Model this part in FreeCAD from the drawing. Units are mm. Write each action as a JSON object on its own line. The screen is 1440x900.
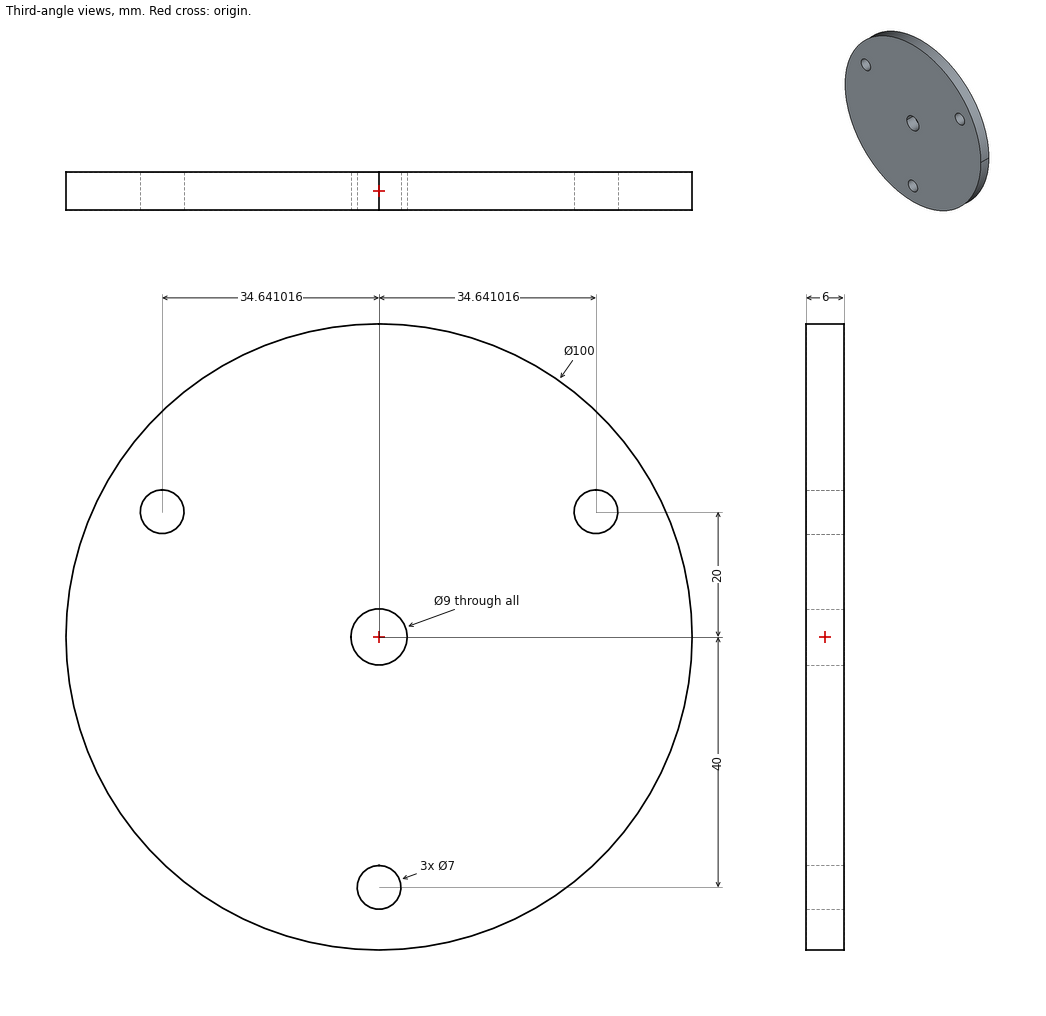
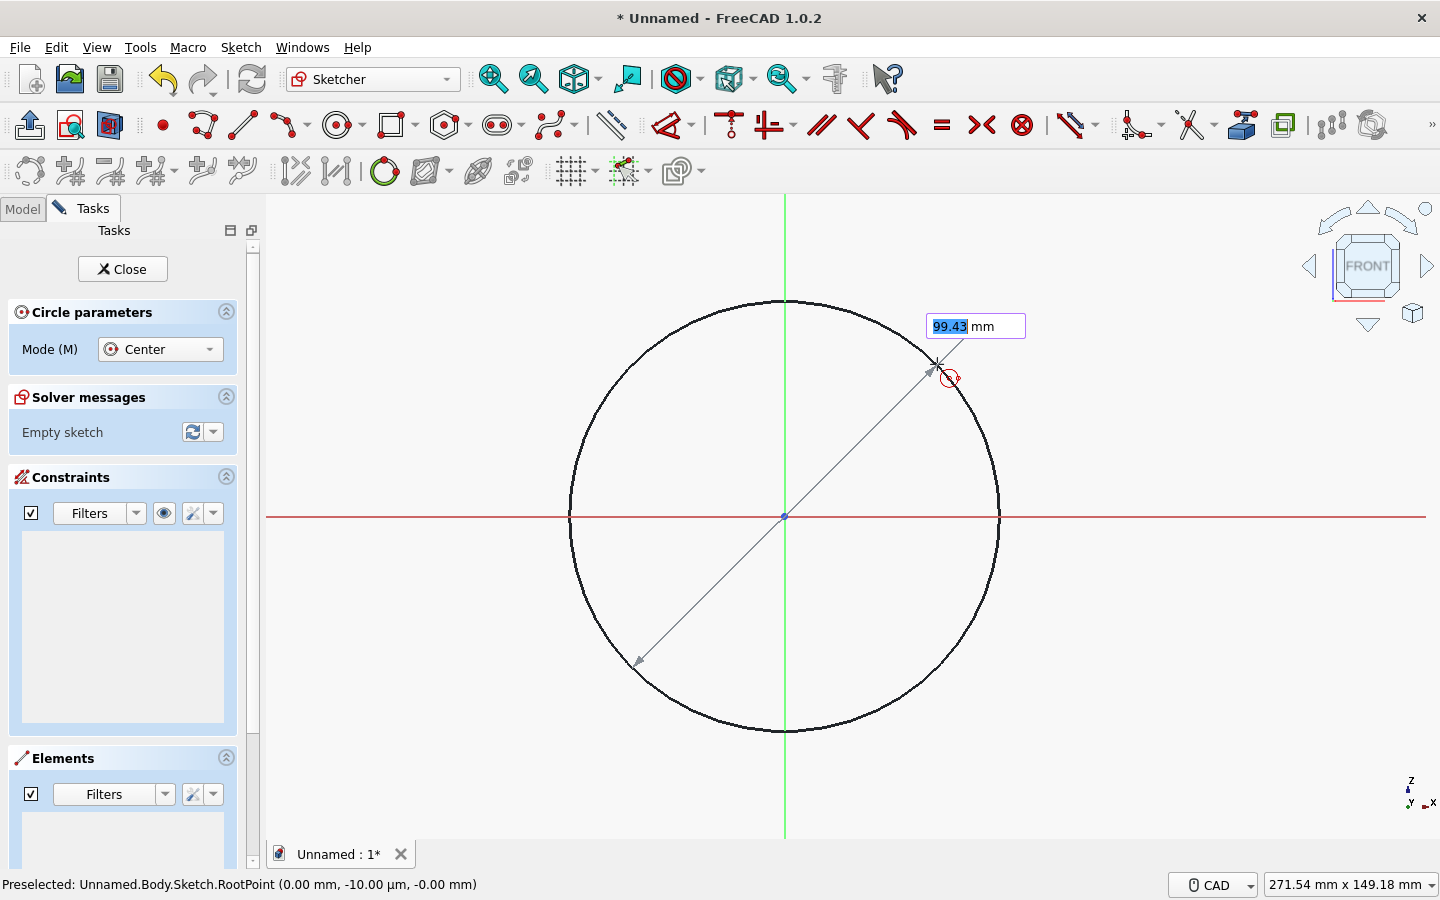
{"action": "type", "text": "100"}
{"action": "key", "text": "Return"}
{"action": "key", "text": "Escape"}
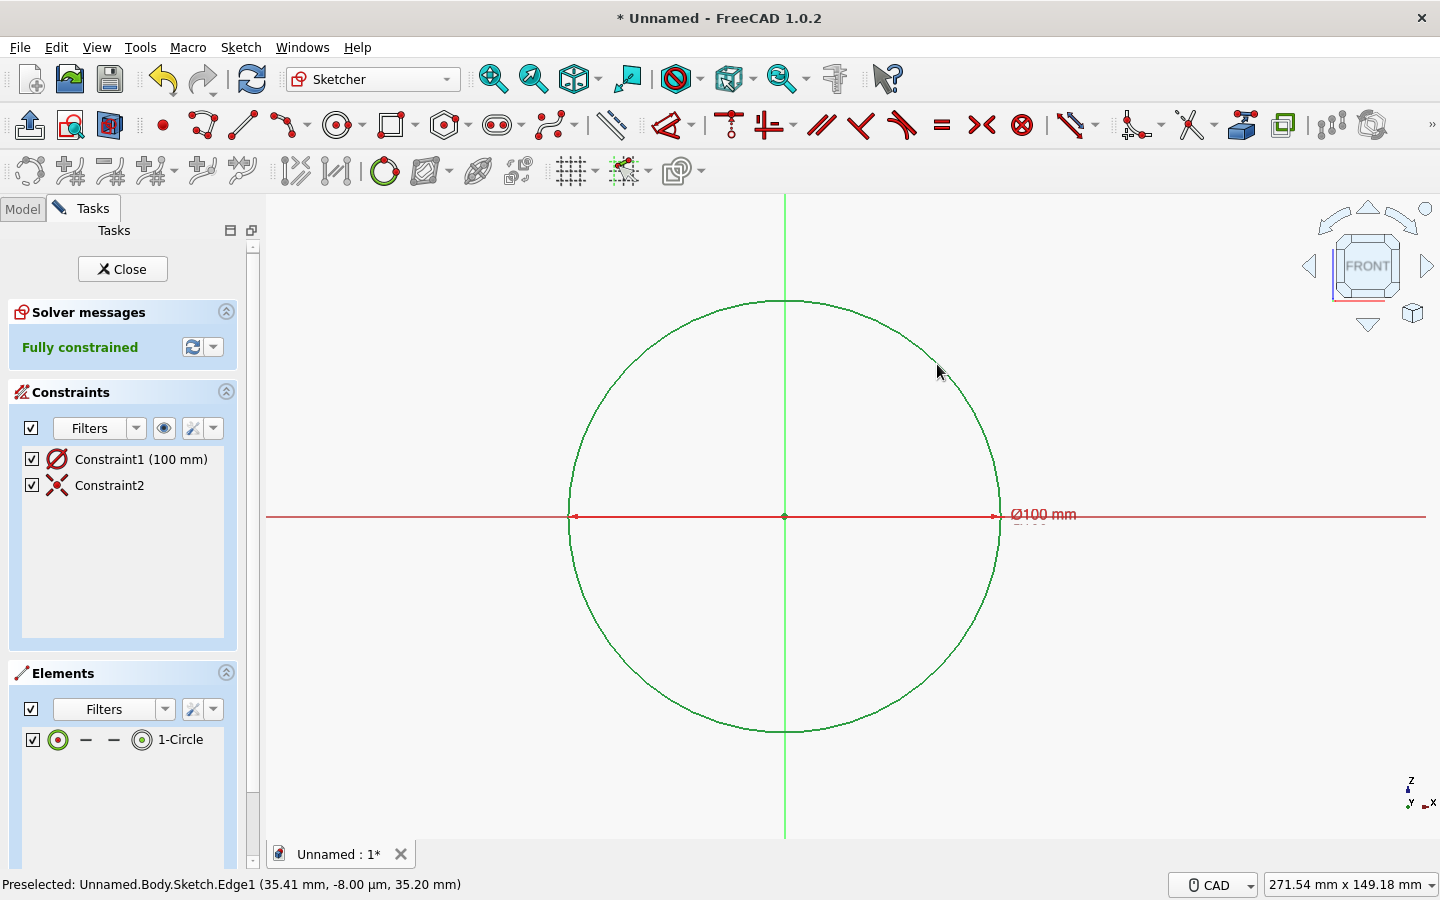
{"action": "left_click", "coordinate": [123, 269]}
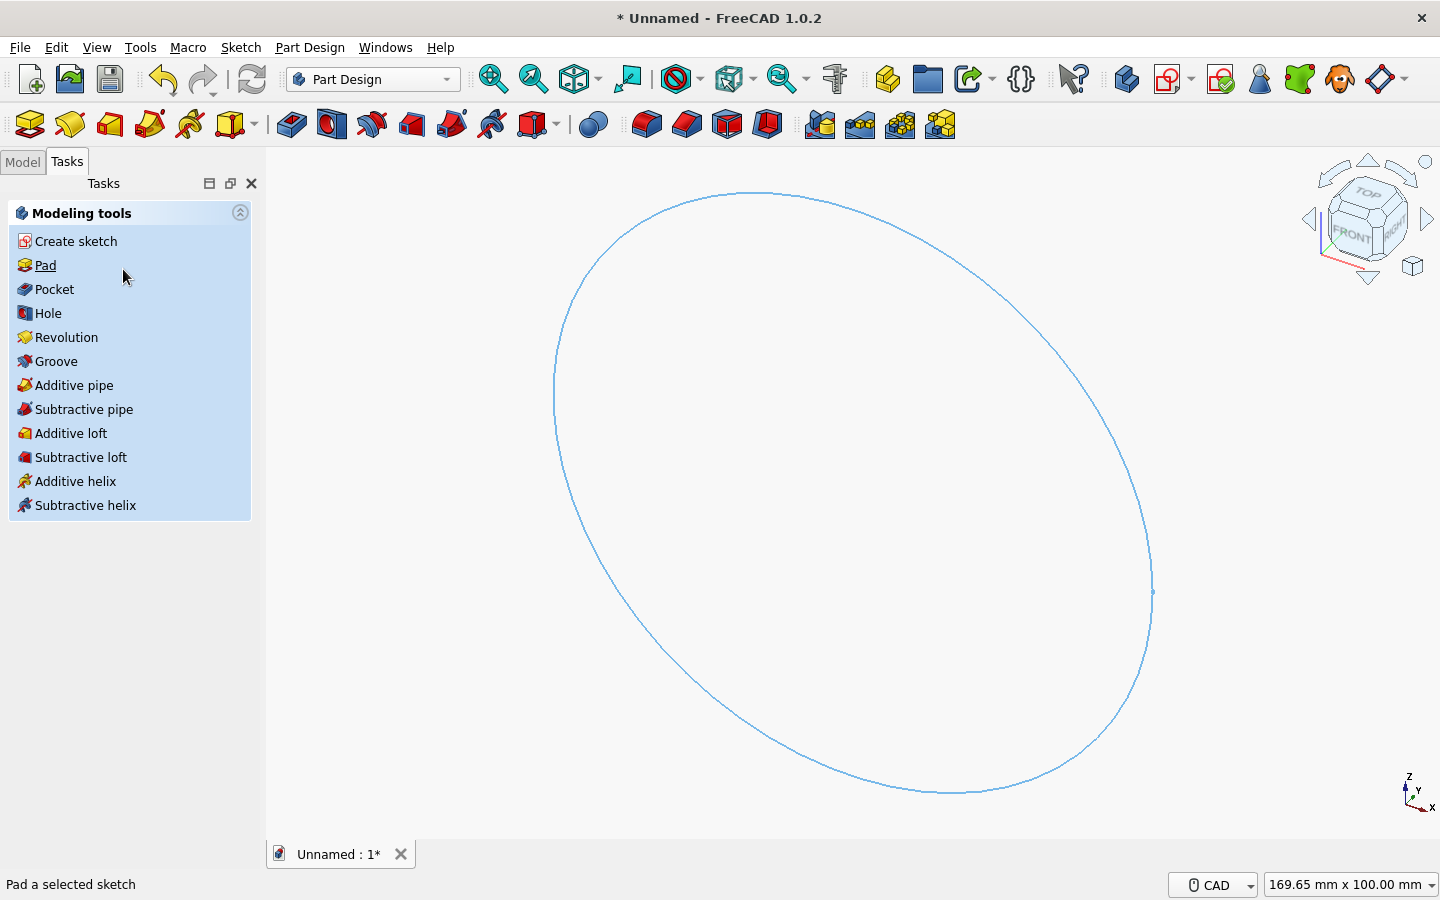
{"action": "left_click", "coordinate": [30, 124]}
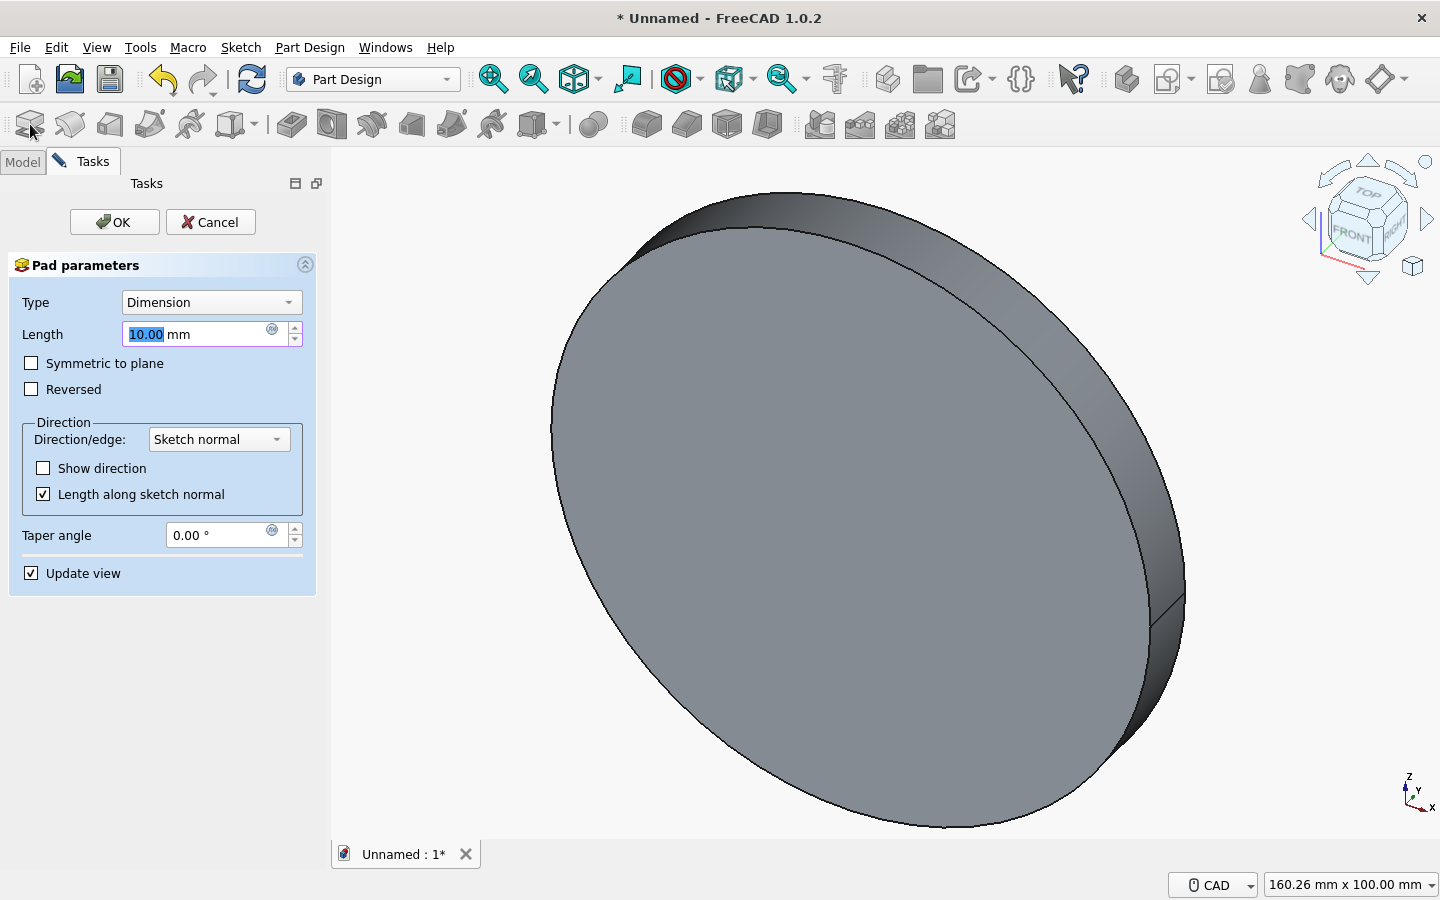
{"action": "type", "text": "6"}
{"action": "key", "text": "Tab"}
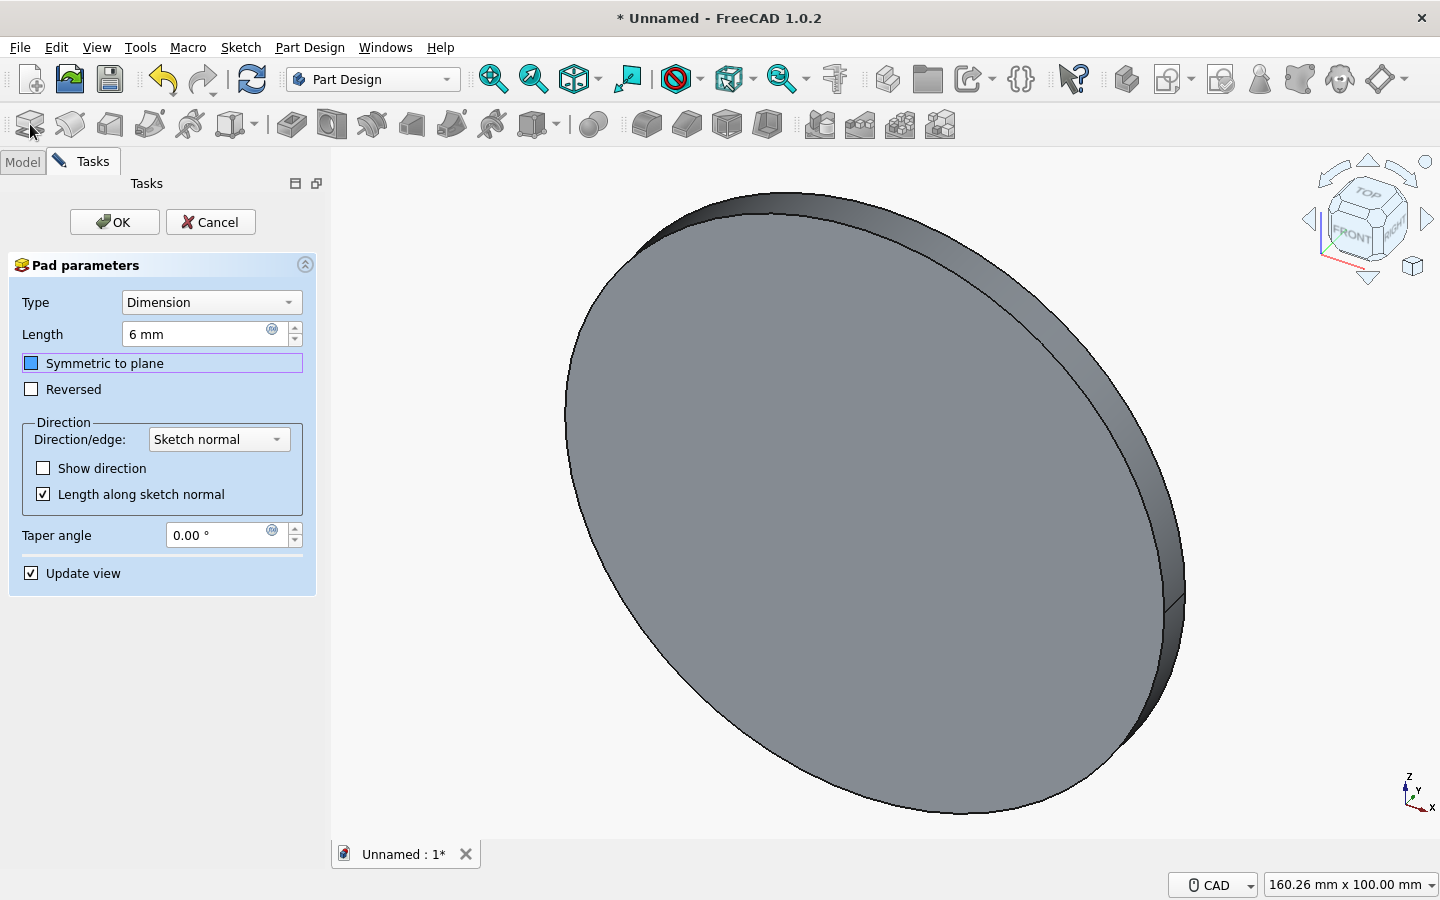
{"action": "left_click", "coordinate": [30, 363]}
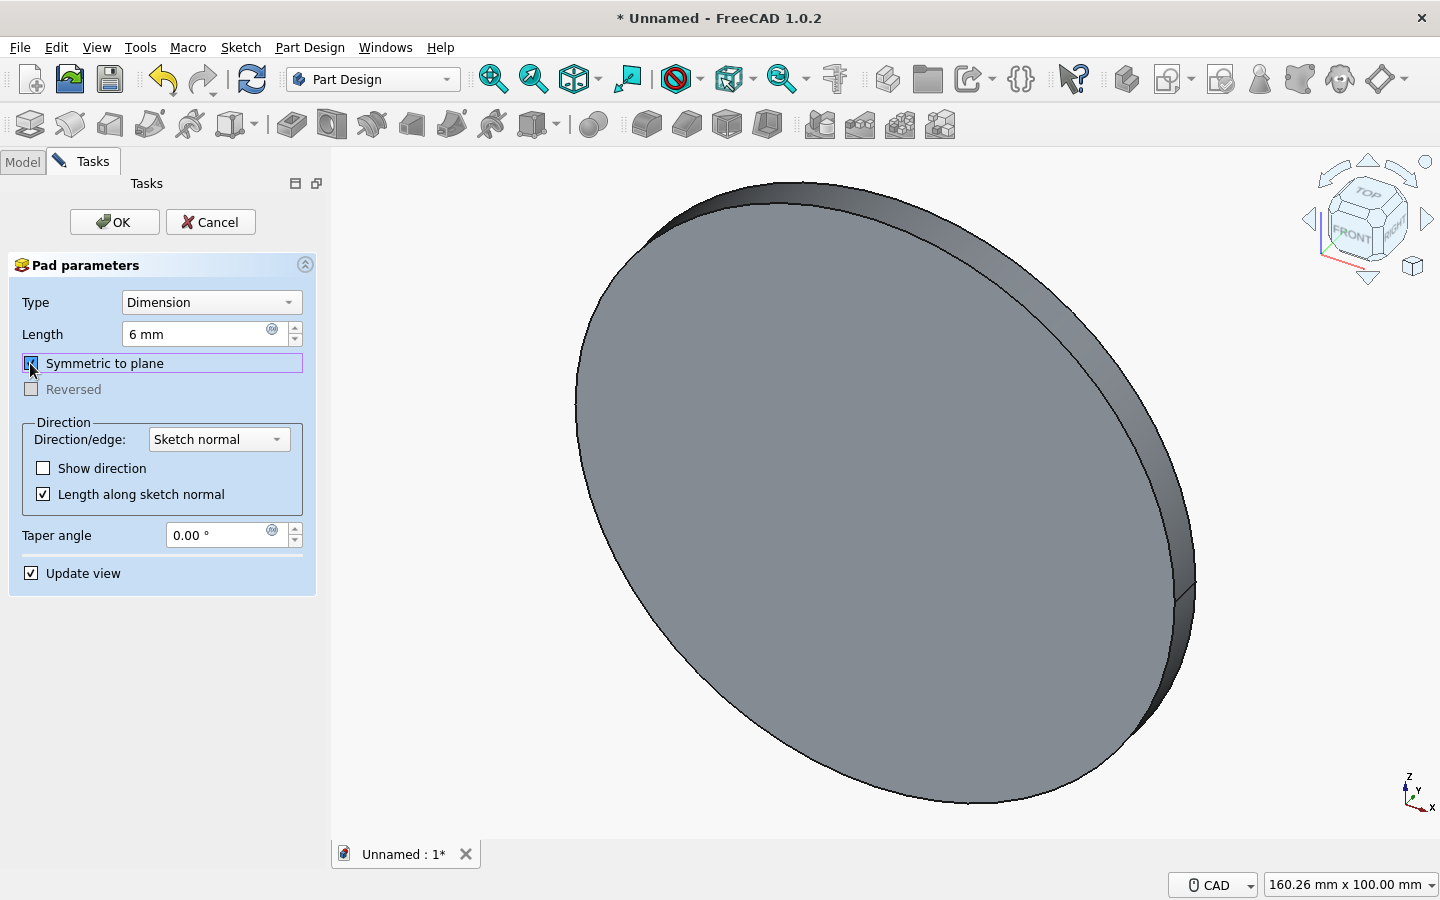
{"action": "left_click", "coordinate": [115, 222]}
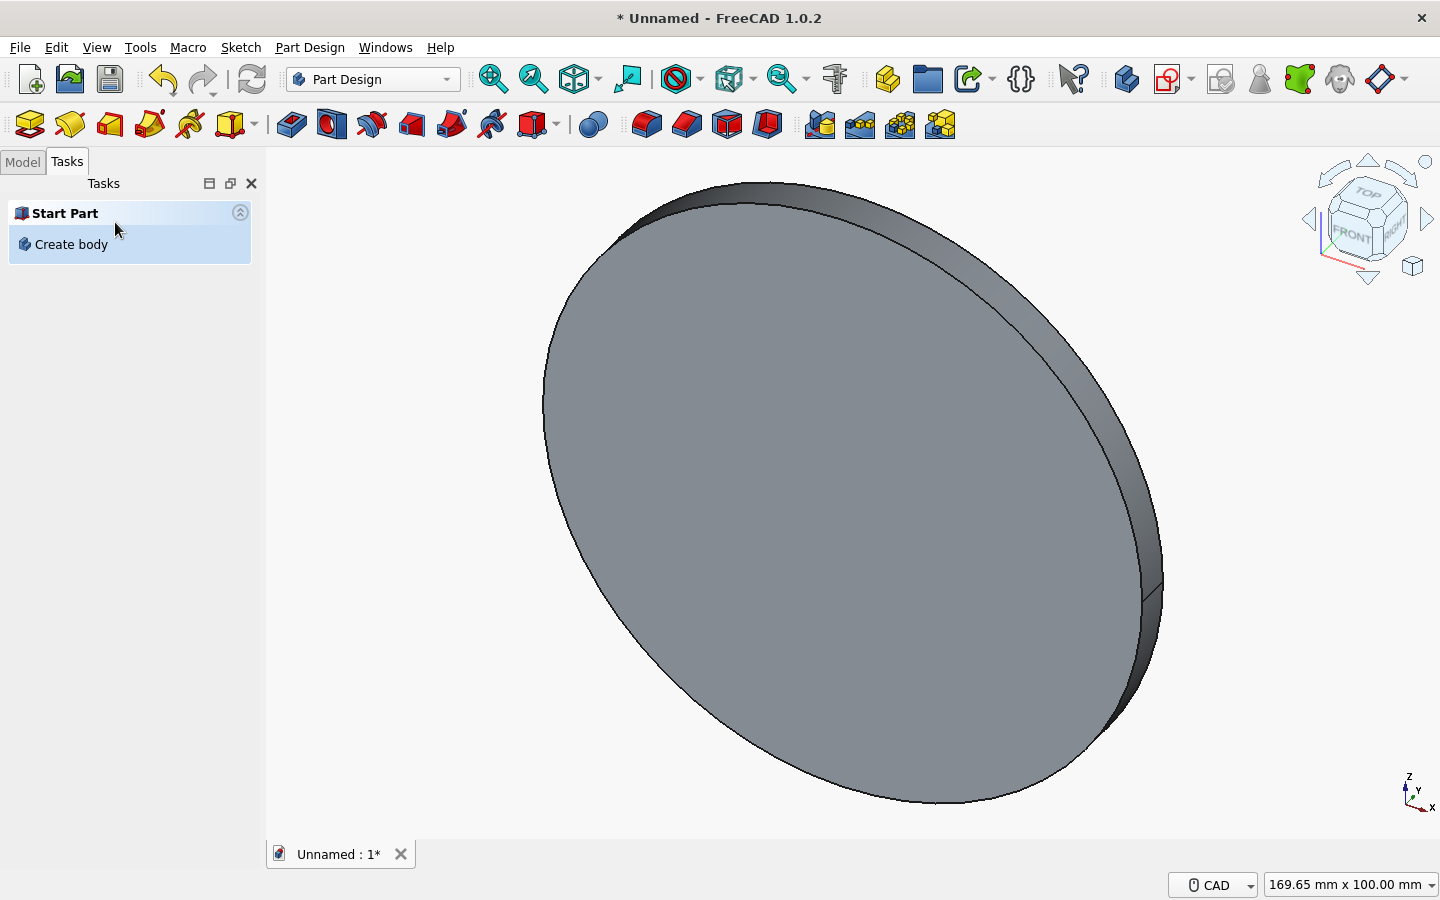
{"action": "left_click", "coordinate": [494, 80]}